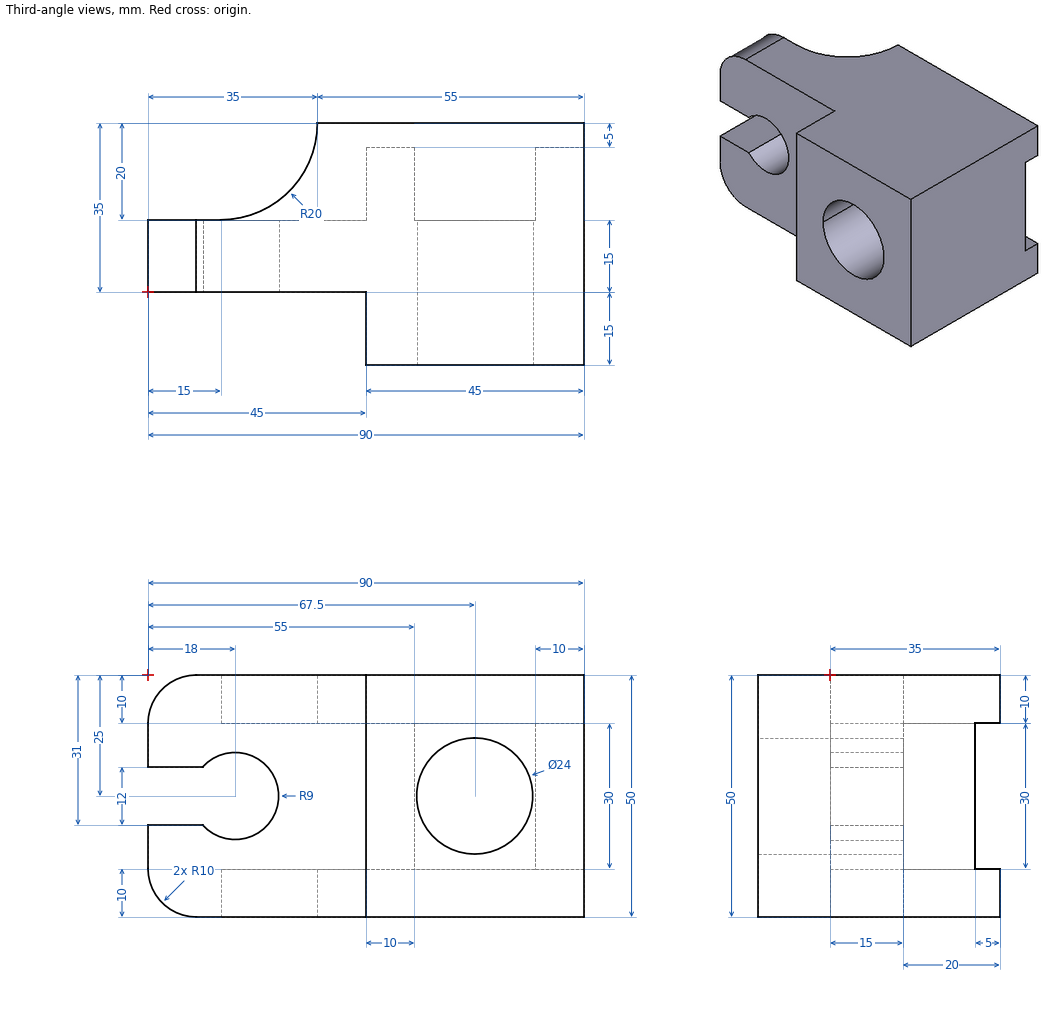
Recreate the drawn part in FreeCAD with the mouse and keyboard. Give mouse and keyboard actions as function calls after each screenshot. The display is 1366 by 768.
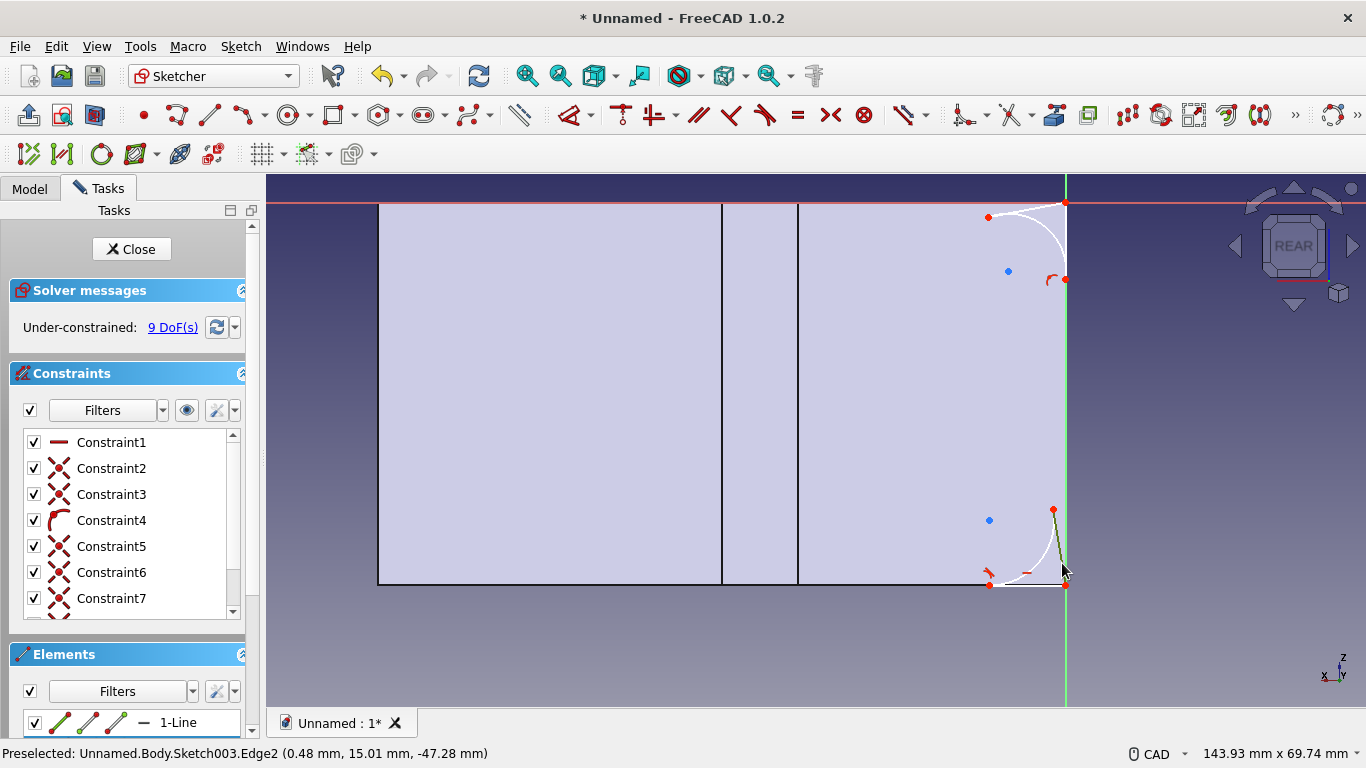
click(1039, 562)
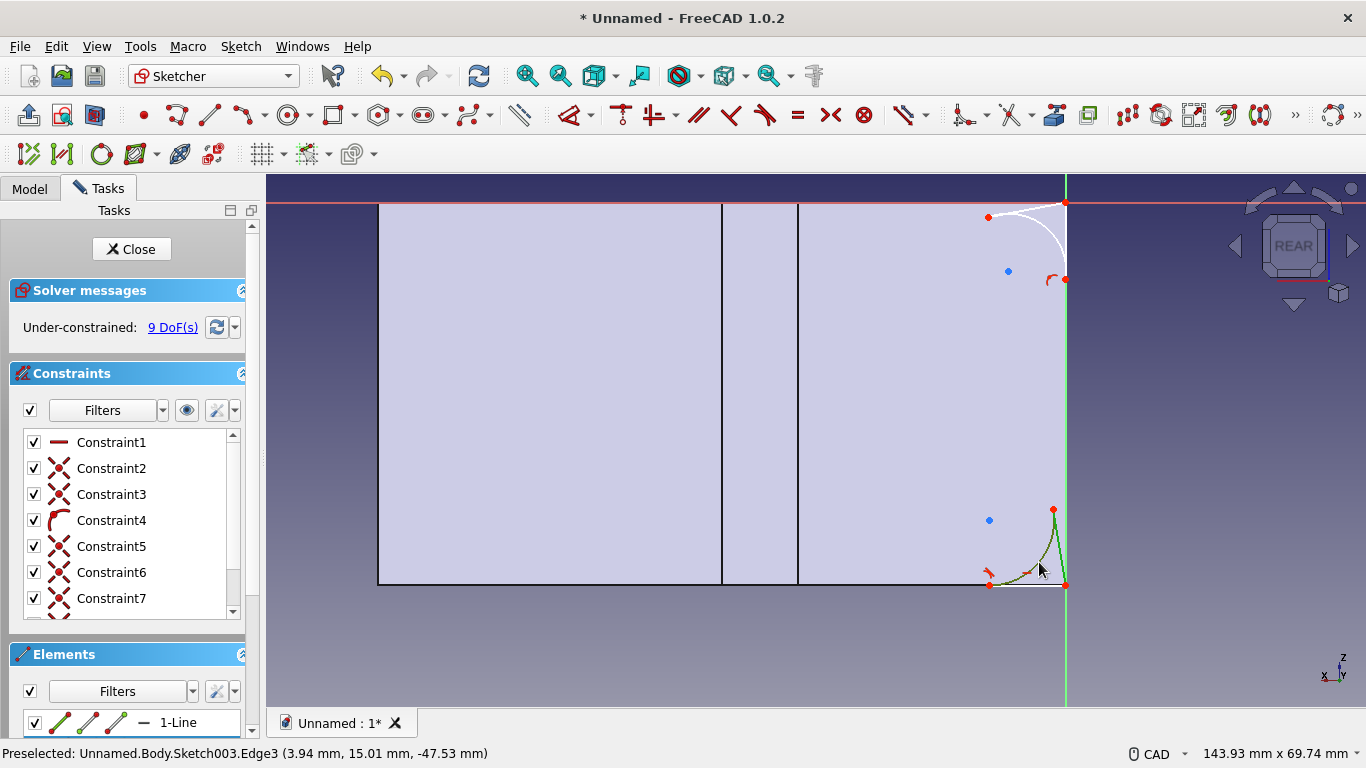
click(765, 116)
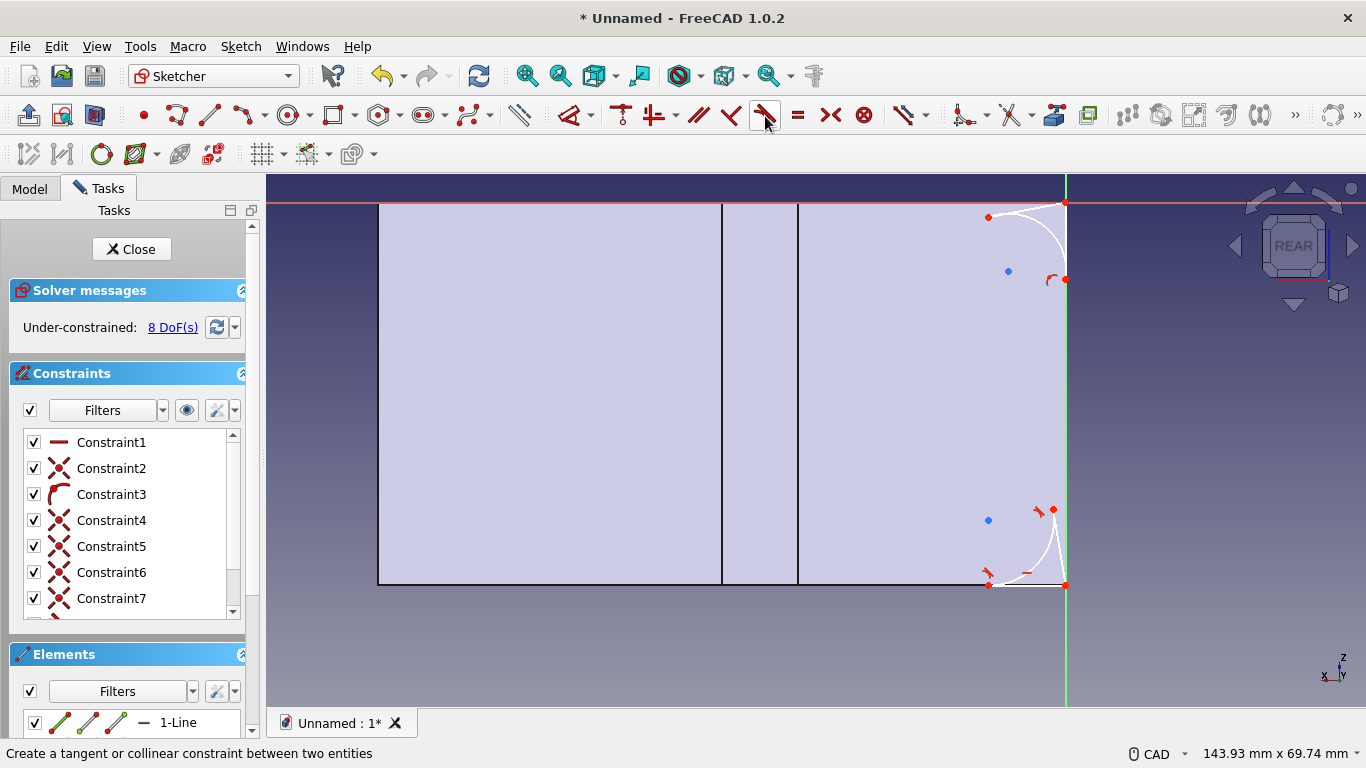
click(1066, 226)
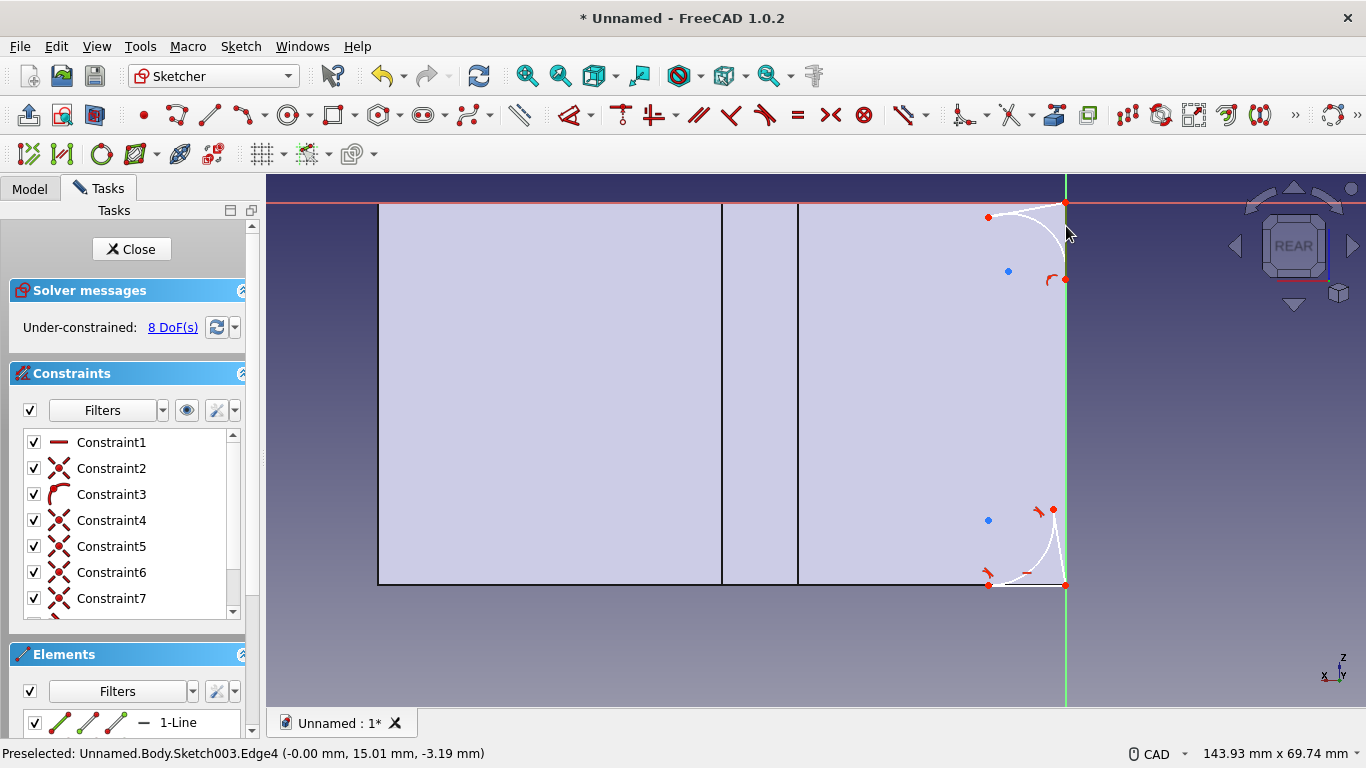
click(1045, 227)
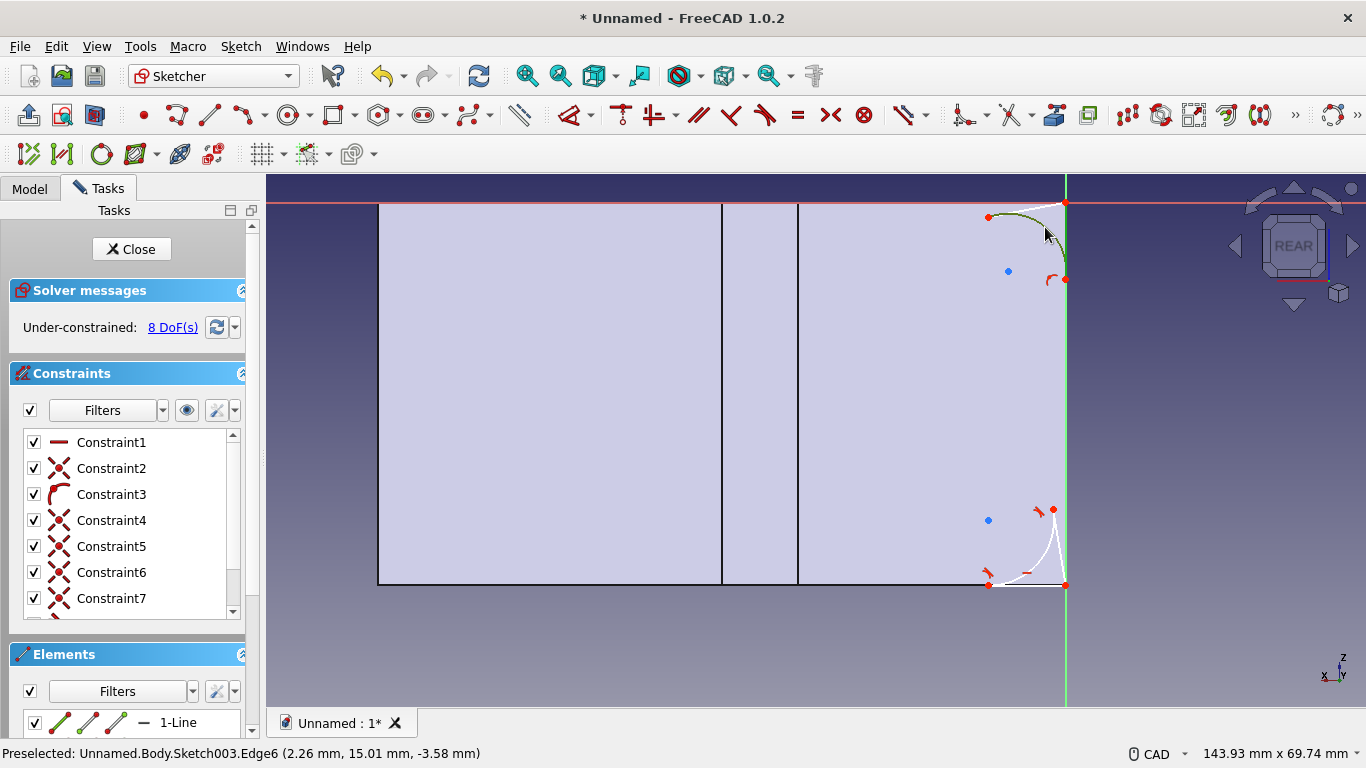
click(765, 116)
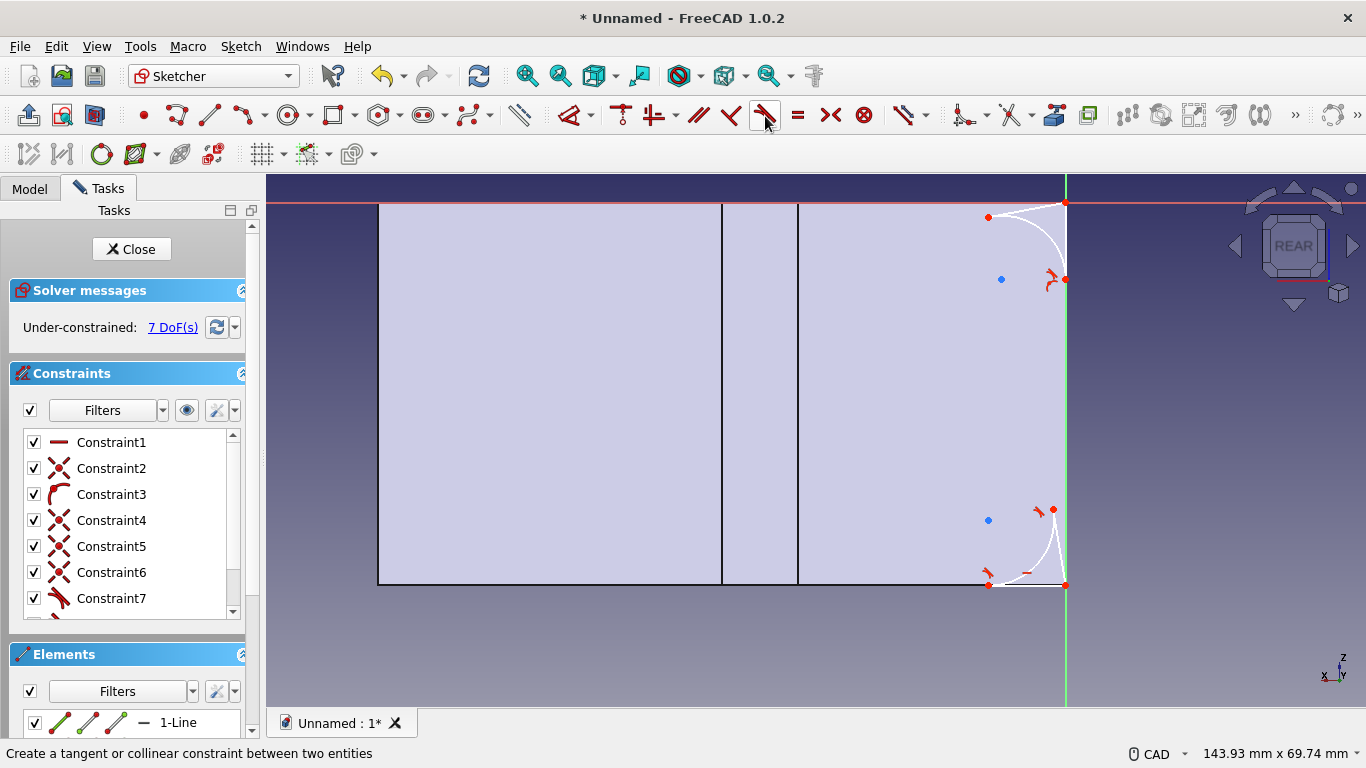
click(1050, 206)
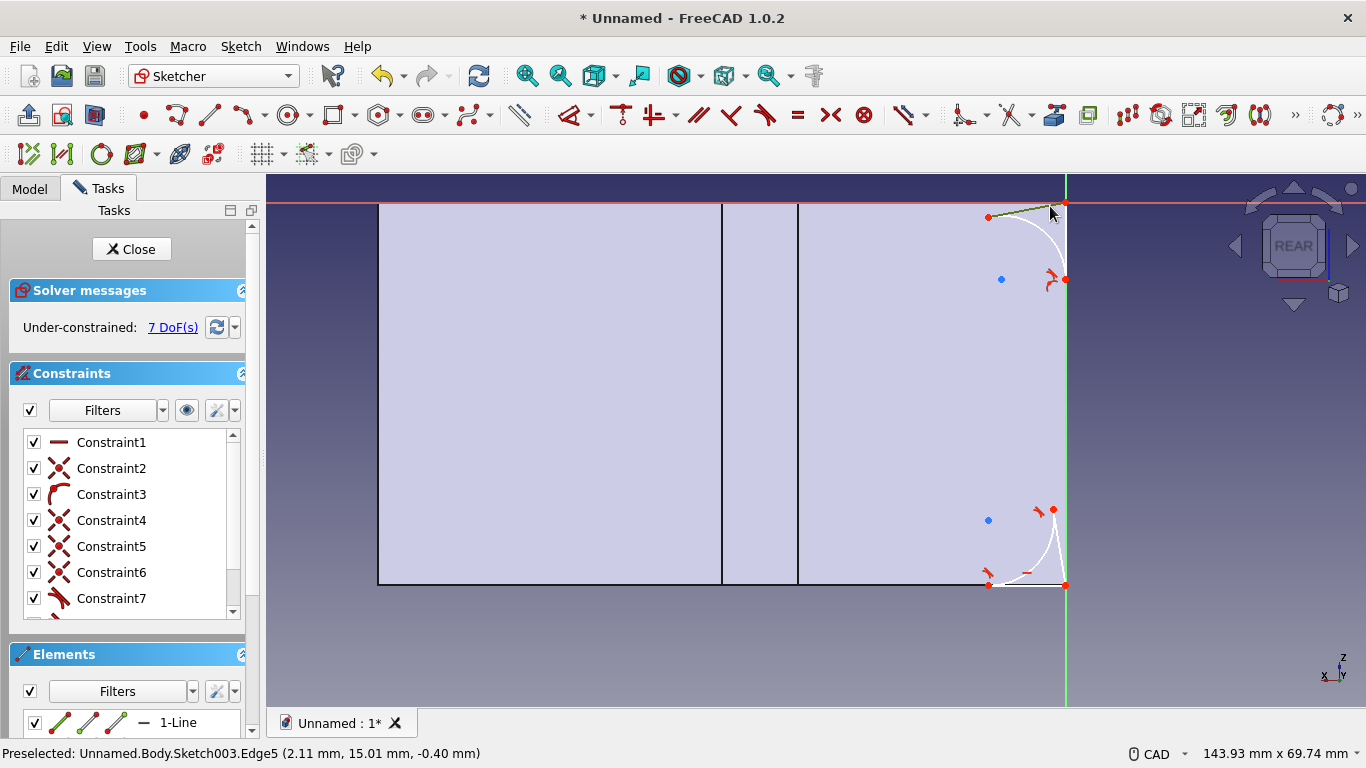
click(1042, 230)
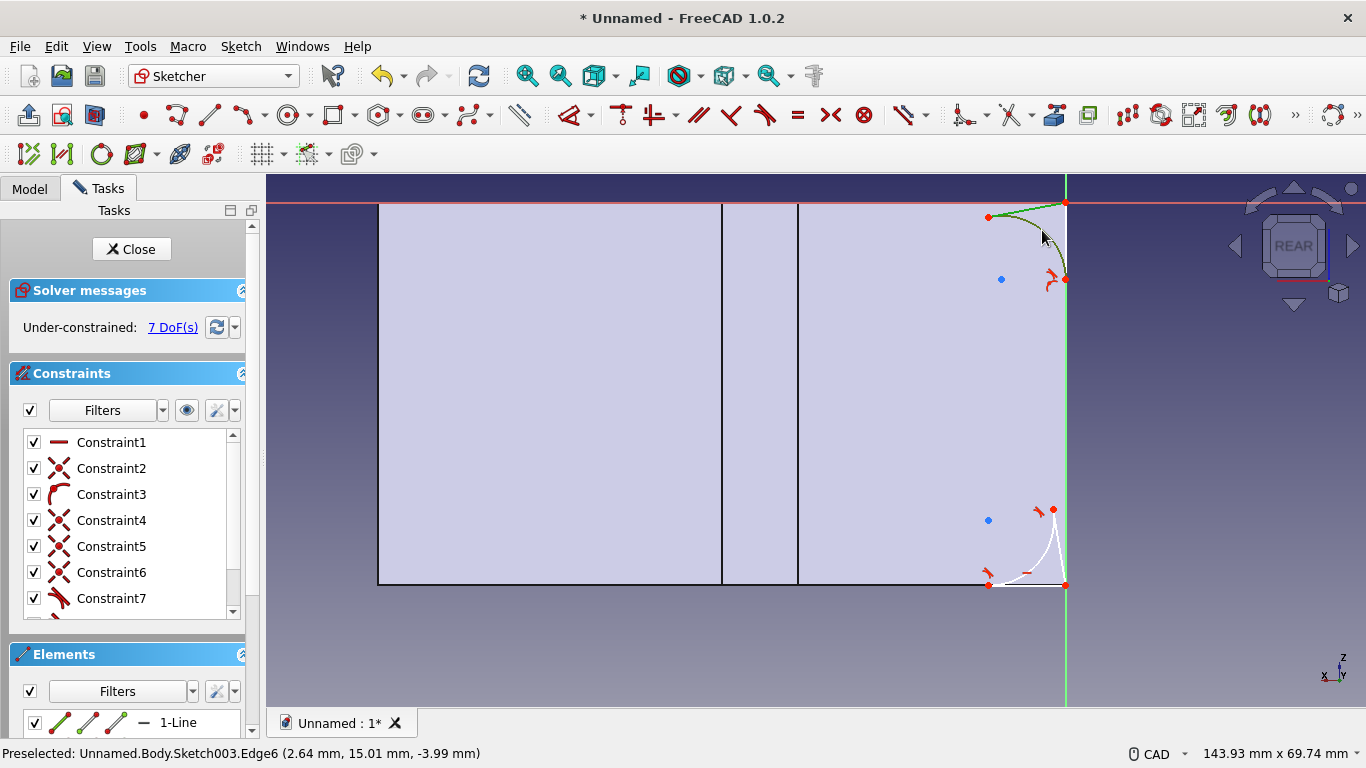
click(765, 116)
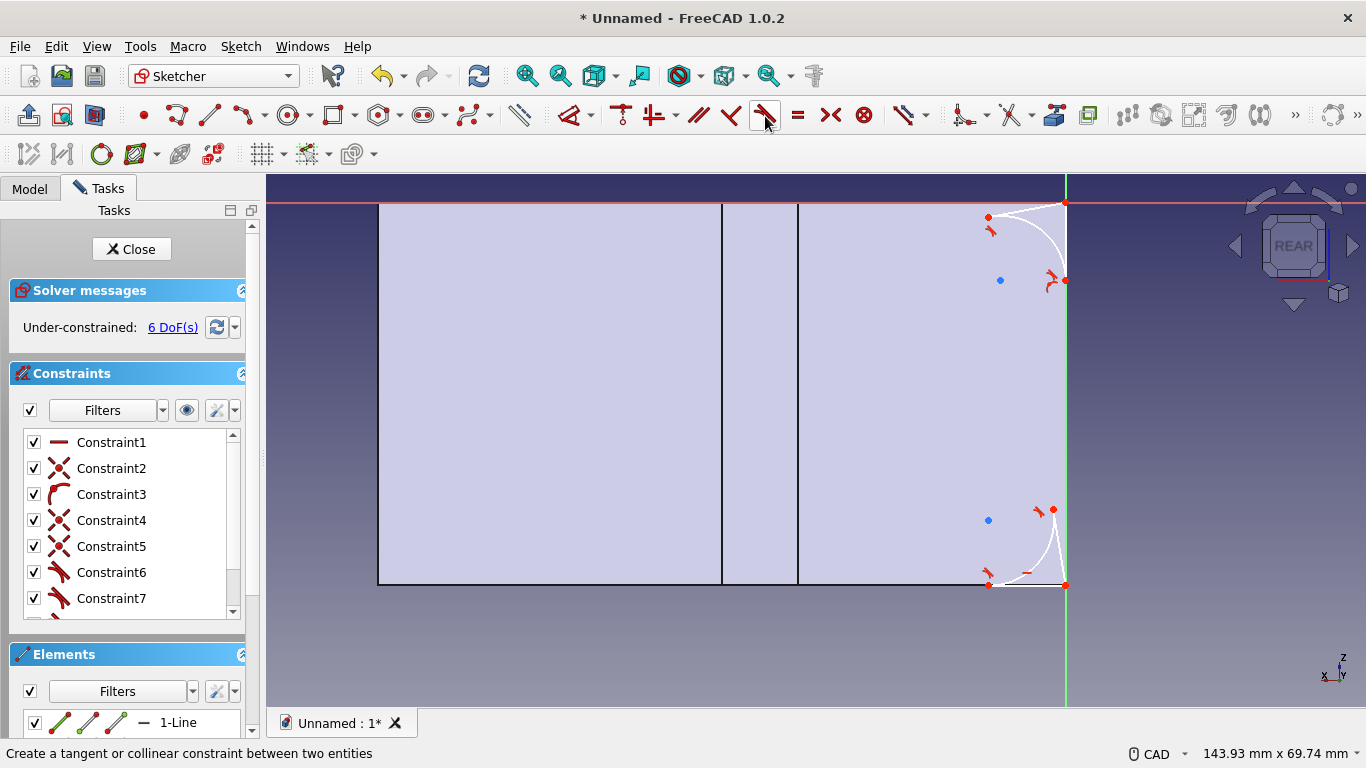
click(1062, 563)